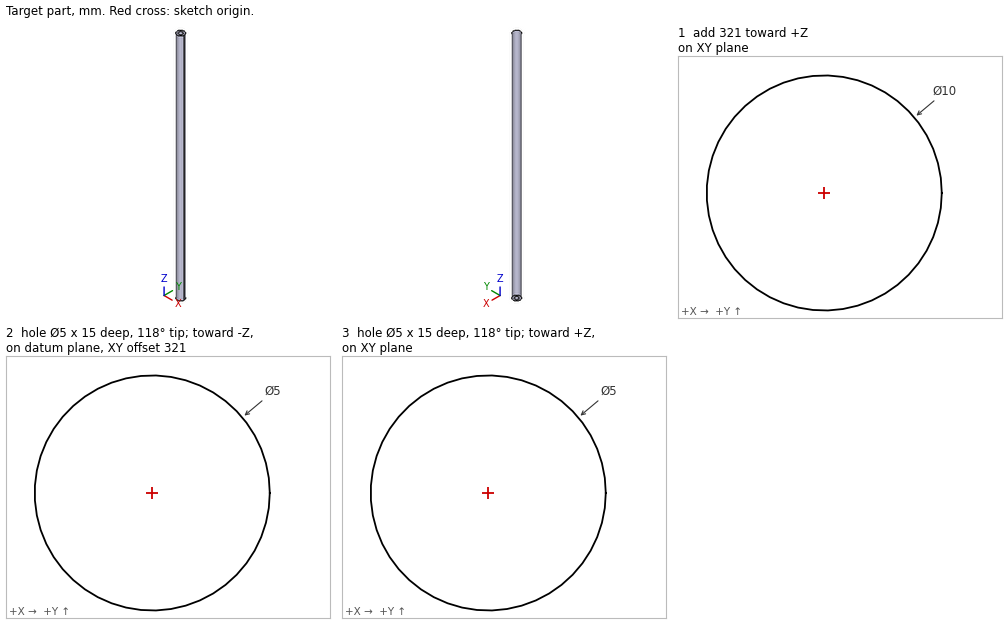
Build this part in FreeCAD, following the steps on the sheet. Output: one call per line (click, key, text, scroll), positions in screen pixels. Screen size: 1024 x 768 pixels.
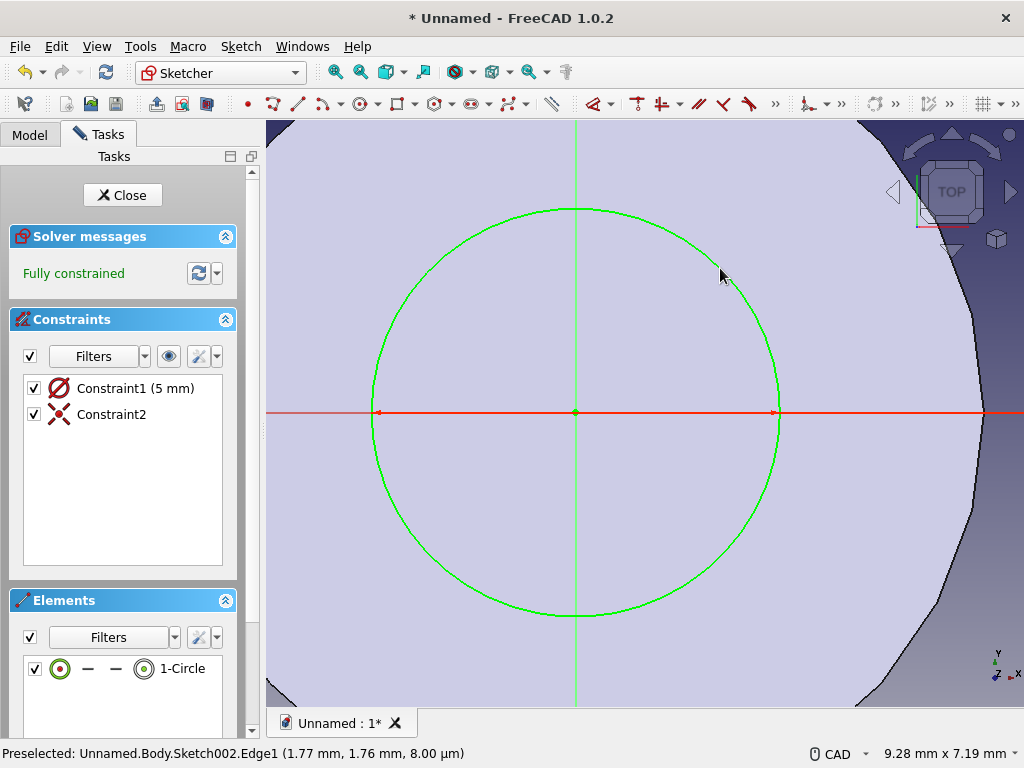
click(123, 195)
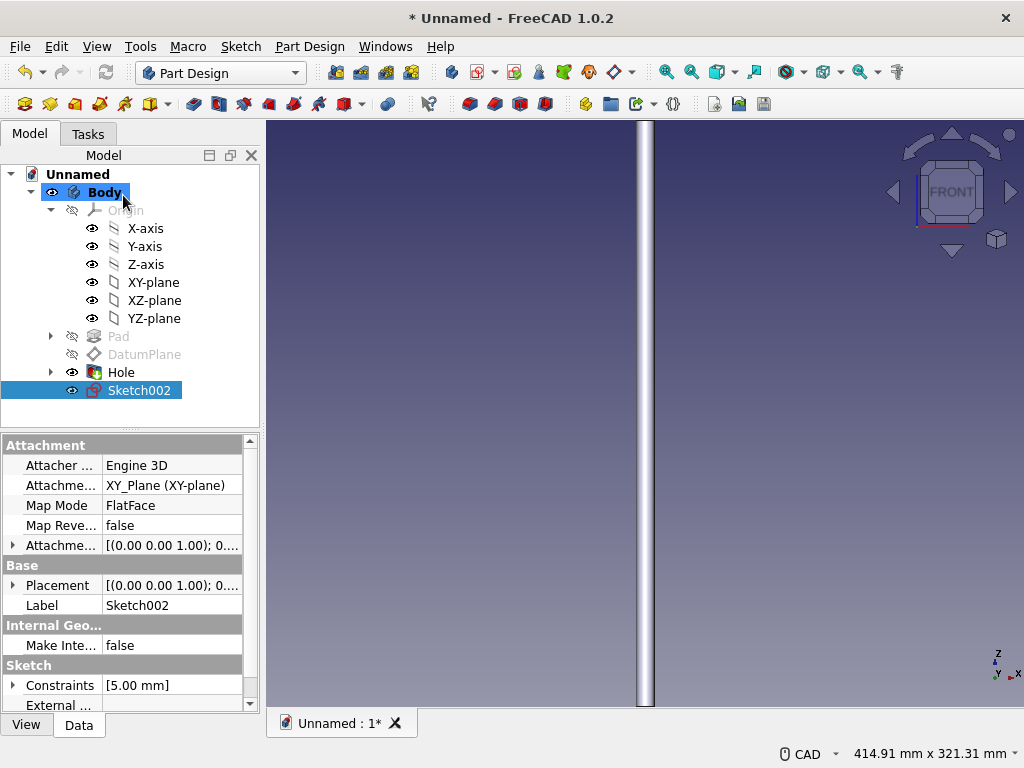
click(219, 104)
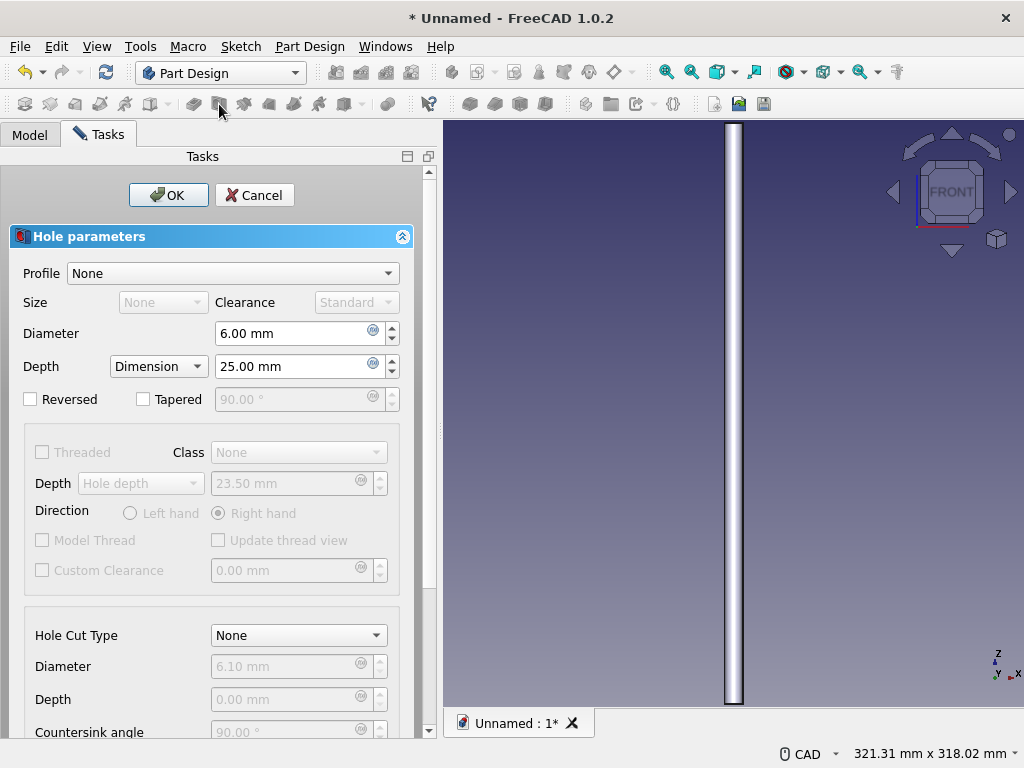
triple_click(300, 334)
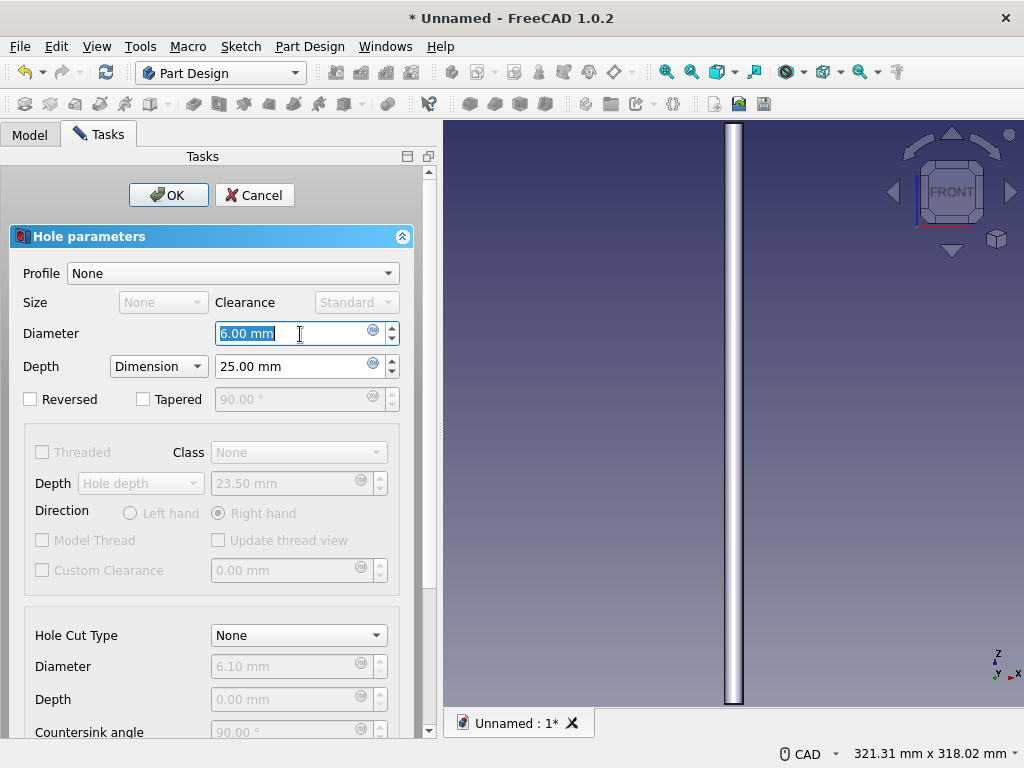
text(5)
key(Tab)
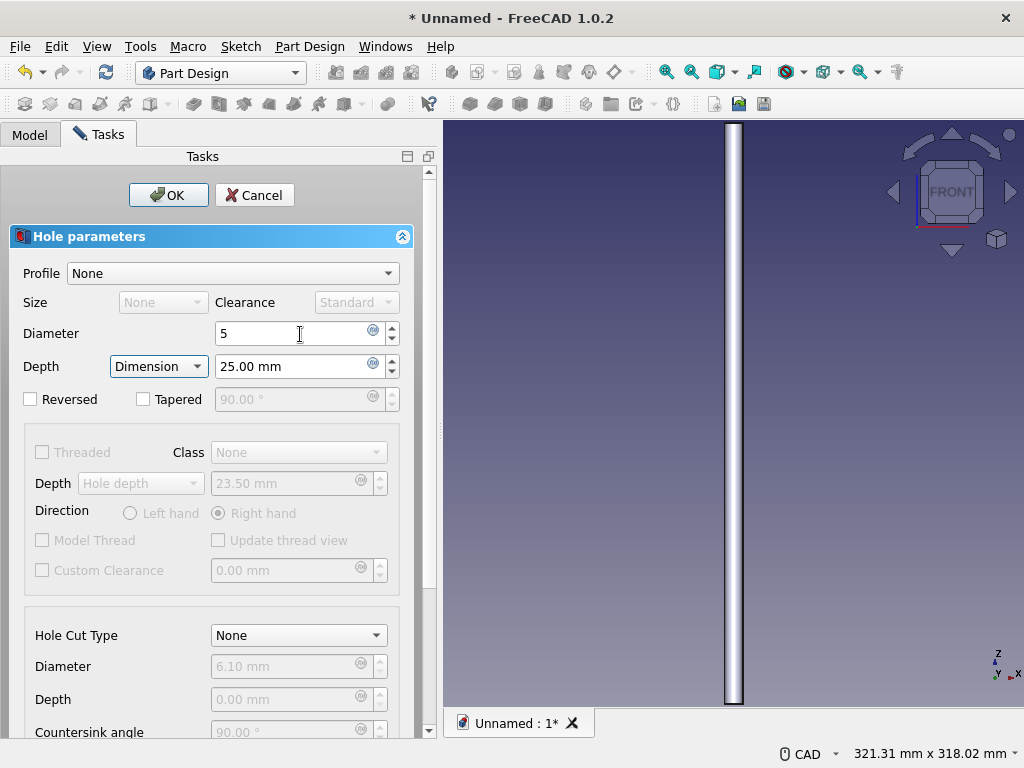
triple_click(300, 366)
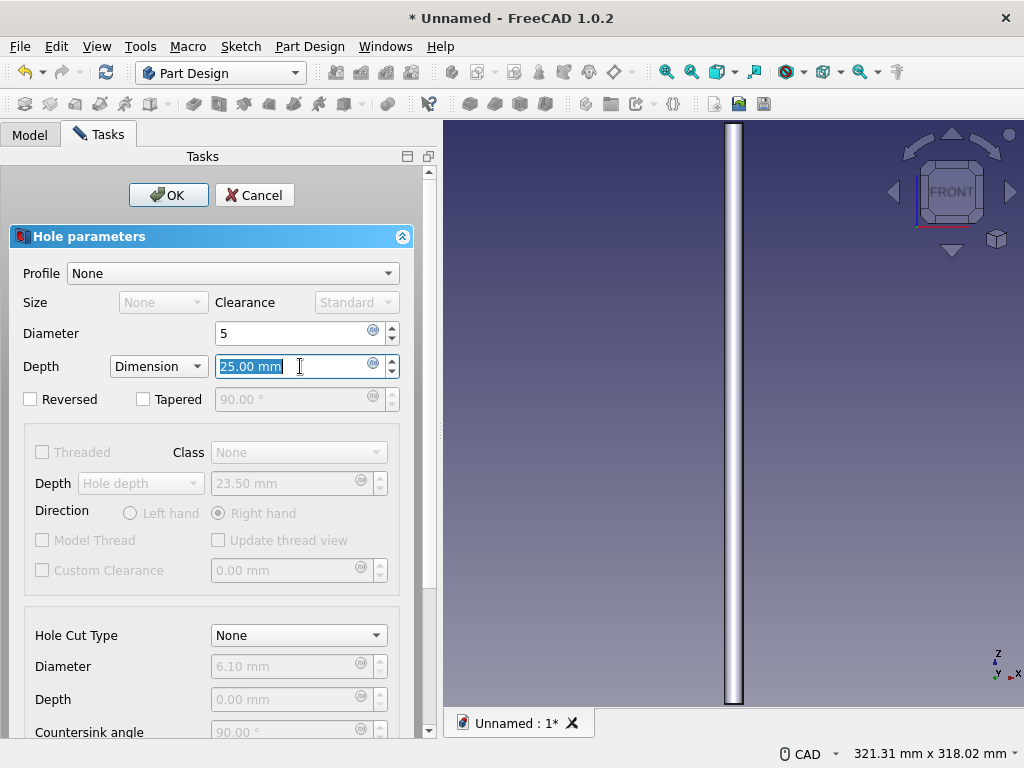
text(15)
key(Tab)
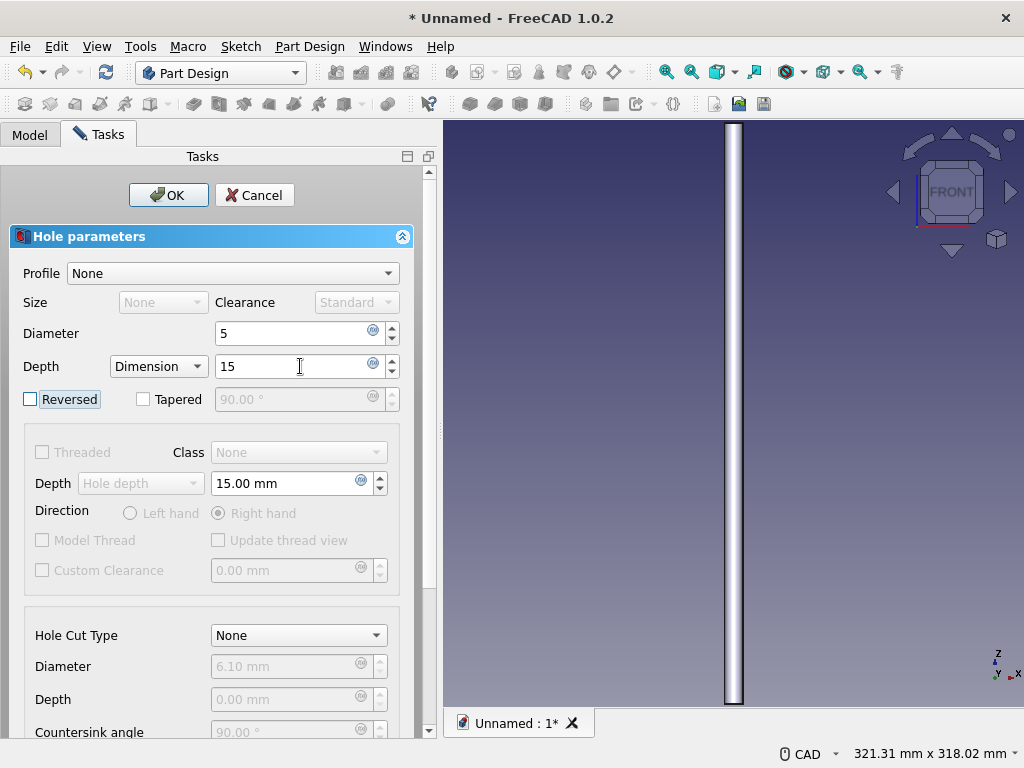
click(31, 399)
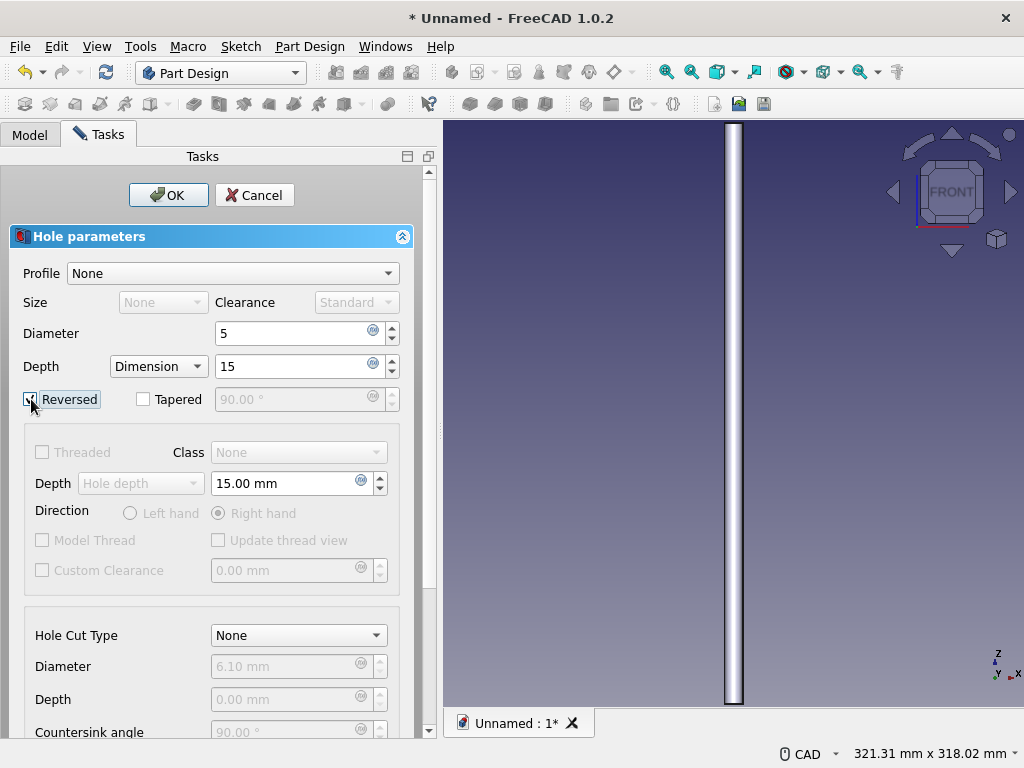
click(169, 195)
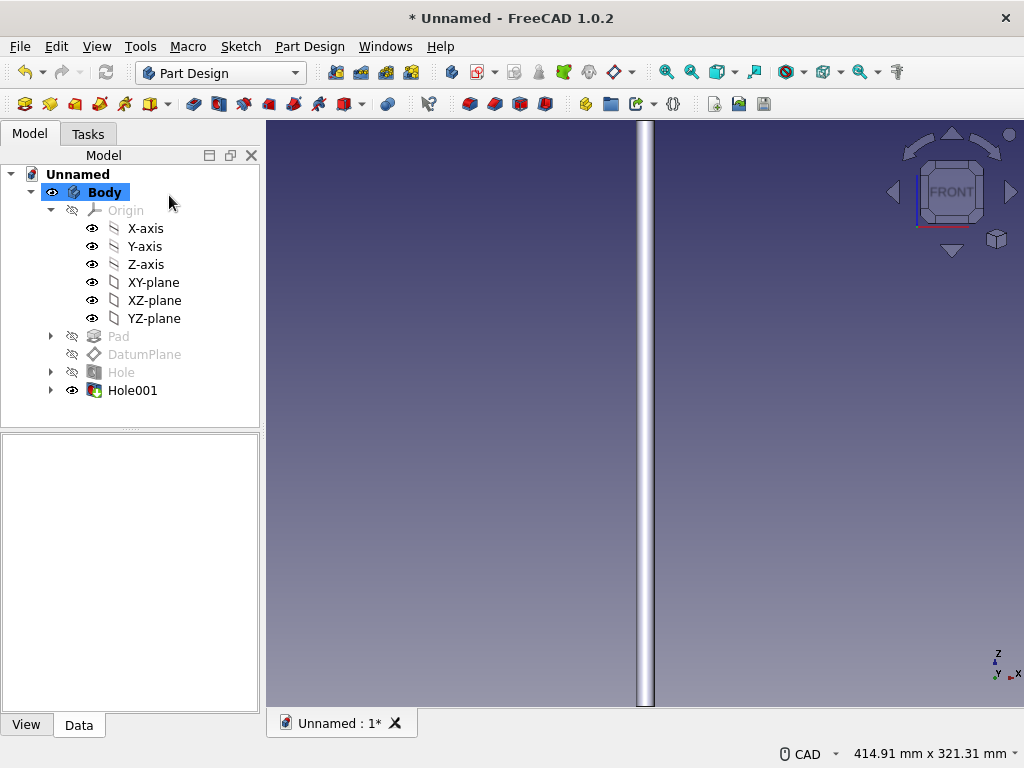
key(0)